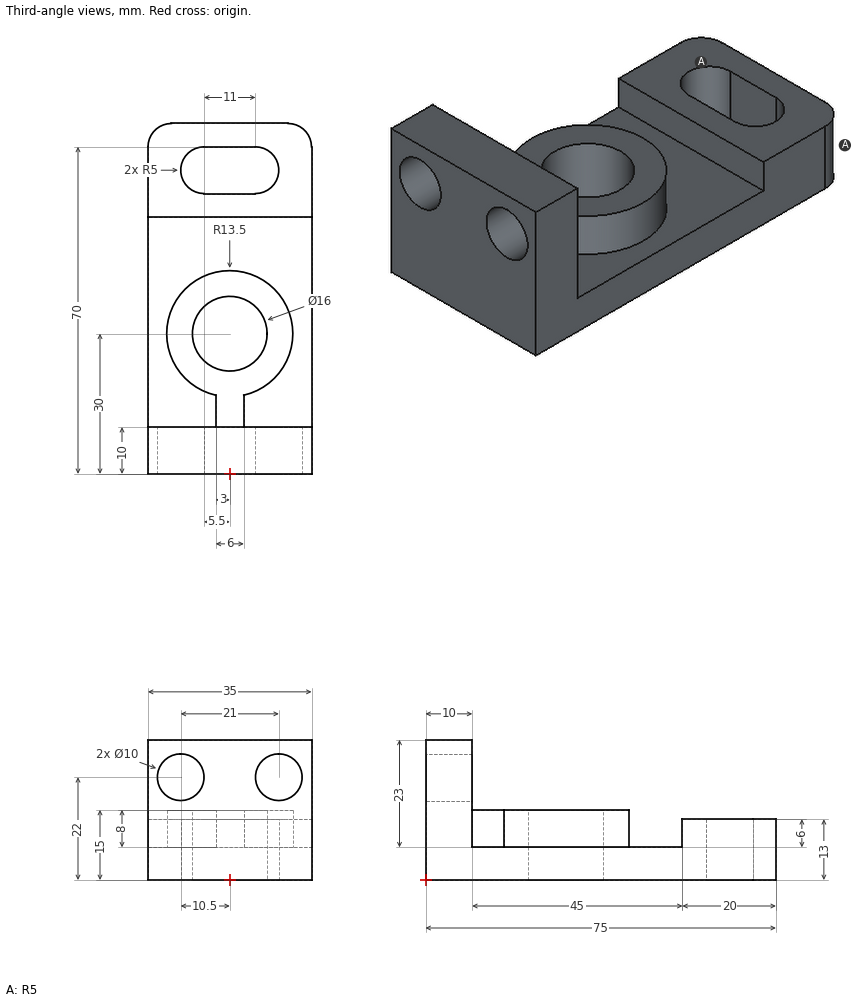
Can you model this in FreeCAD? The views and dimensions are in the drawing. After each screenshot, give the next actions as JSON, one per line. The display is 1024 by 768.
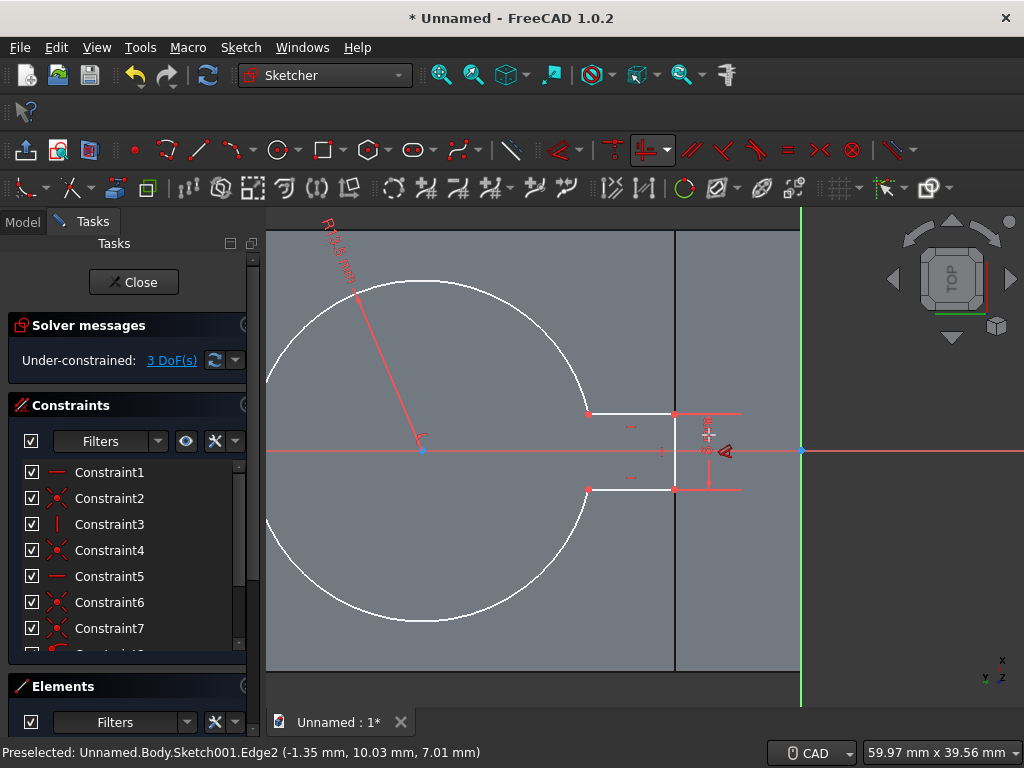
{"action": "left_click", "coordinate": [588, 490]}
{"action": "left_click", "coordinate": [835, 470]}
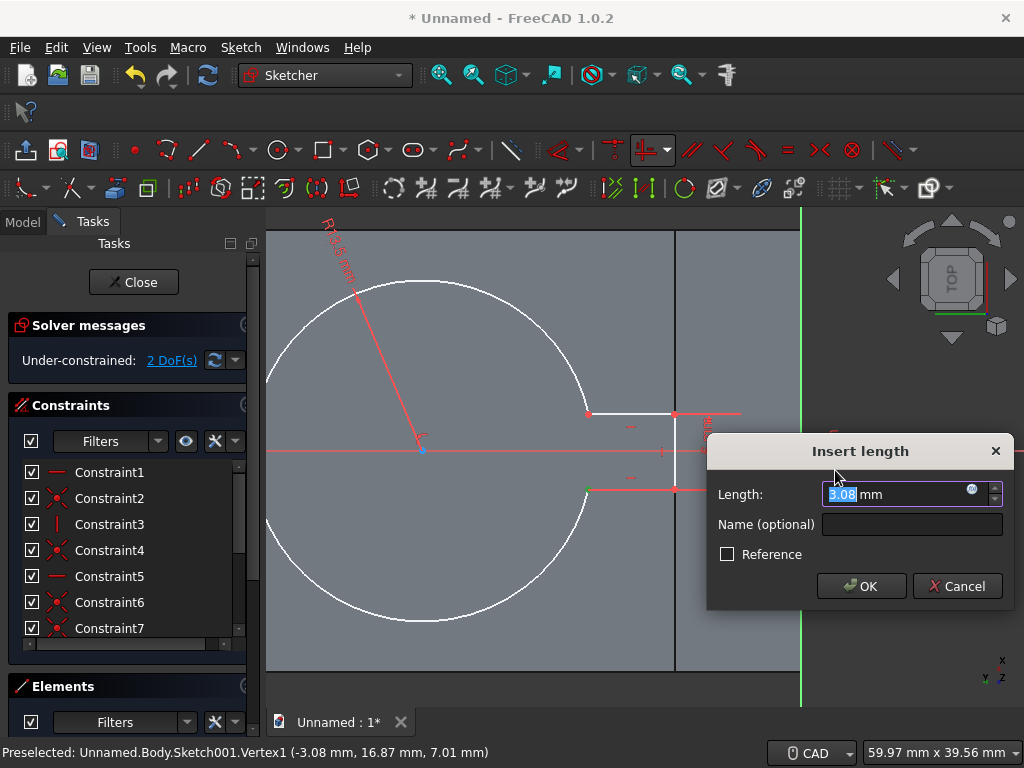
{"action": "type", "text": "3"}
{"action": "key", "text": "Return"}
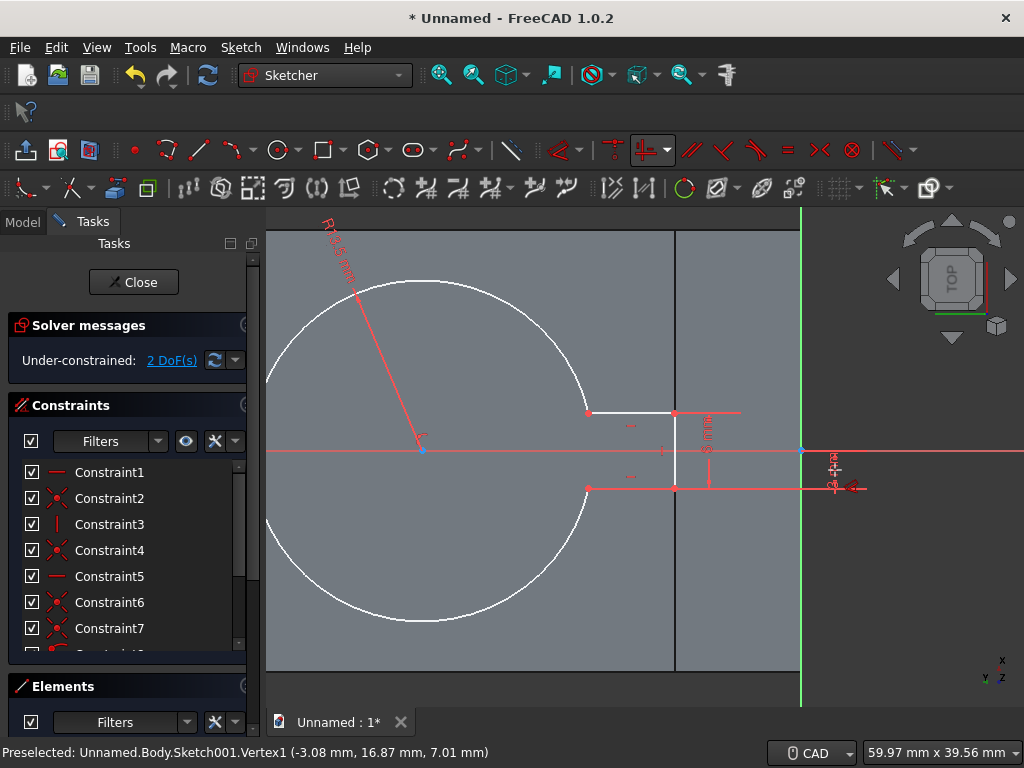
{"action": "left_click", "coordinate": [675, 489]}
{"action": "left_click", "coordinate": [738, 523]}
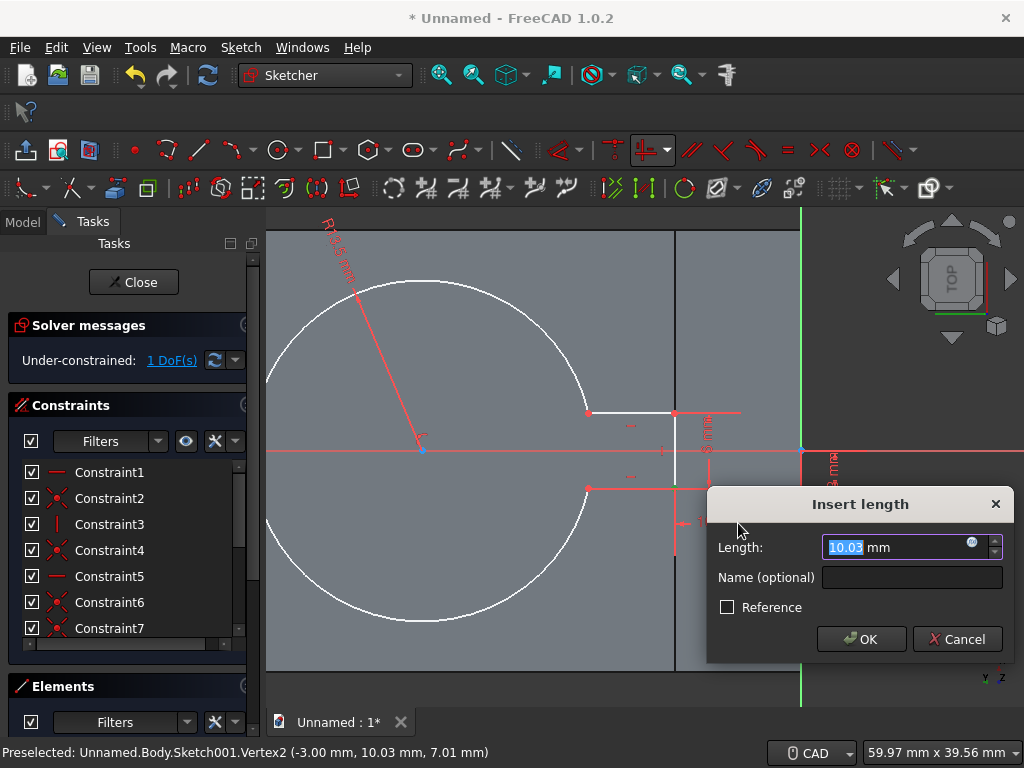
{"action": "type", "text": "10"}
{"action": "key", "text": "Return"}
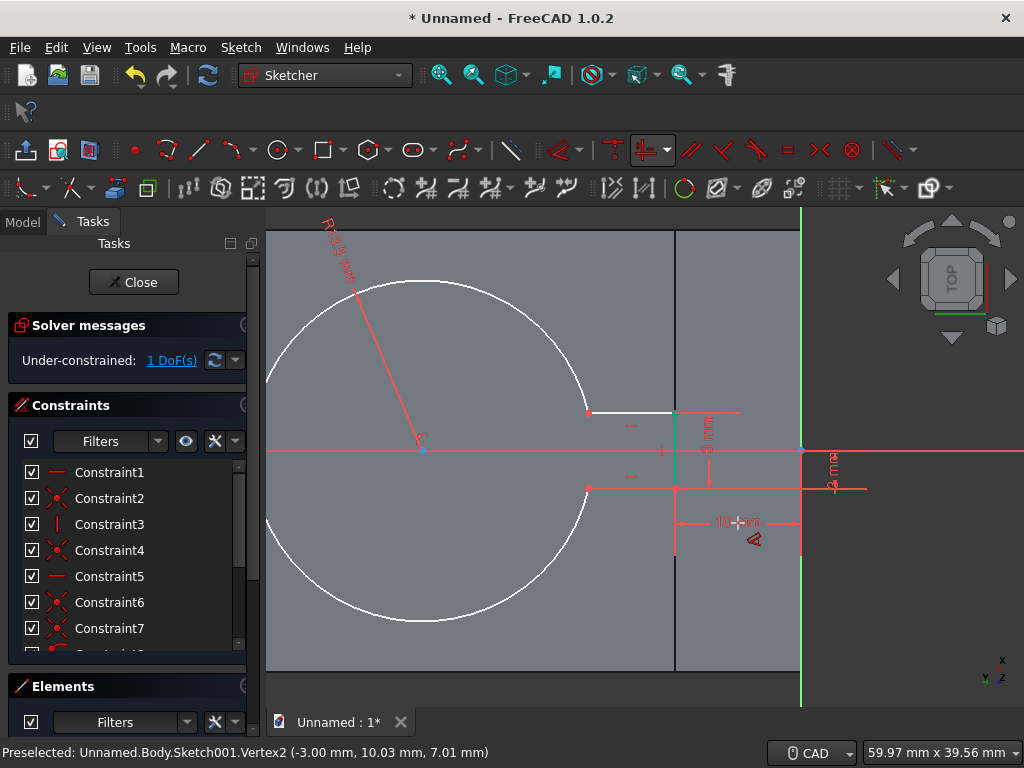
{"action": "left_click", "coordinate": [422, 451]}
{"action": "left_click", "coordinate": [525, 417]}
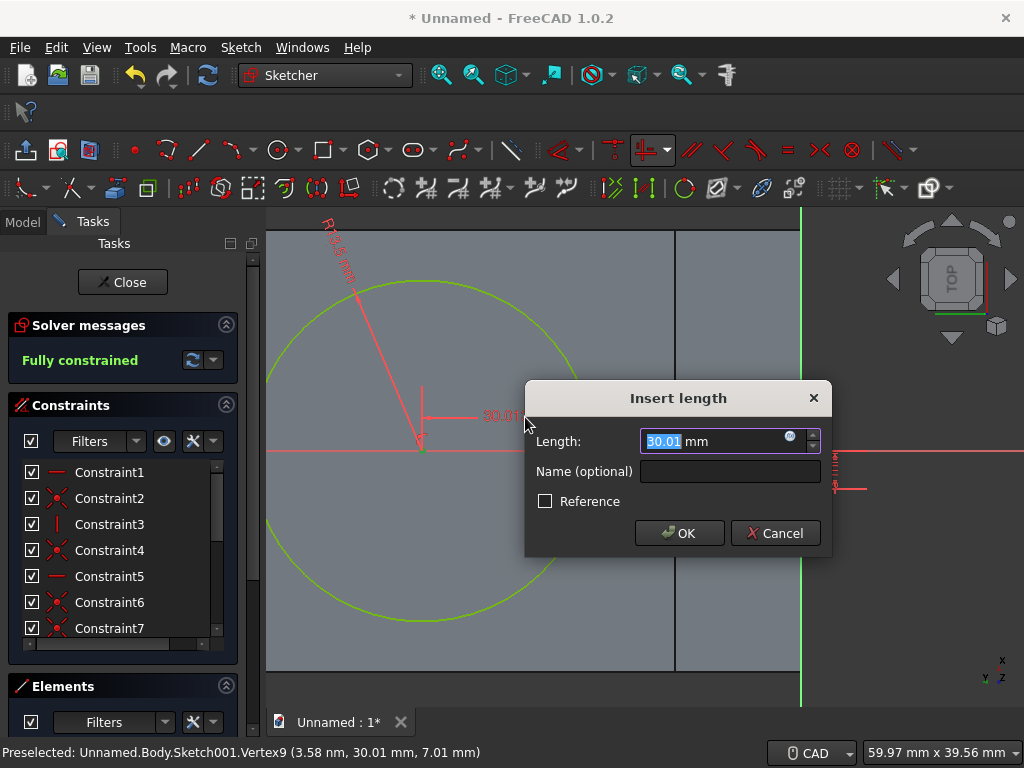
{"action": "type", "text": "30"}
{"action": "key", "text": "Return"}
{"action": "key", "text": "Escape"}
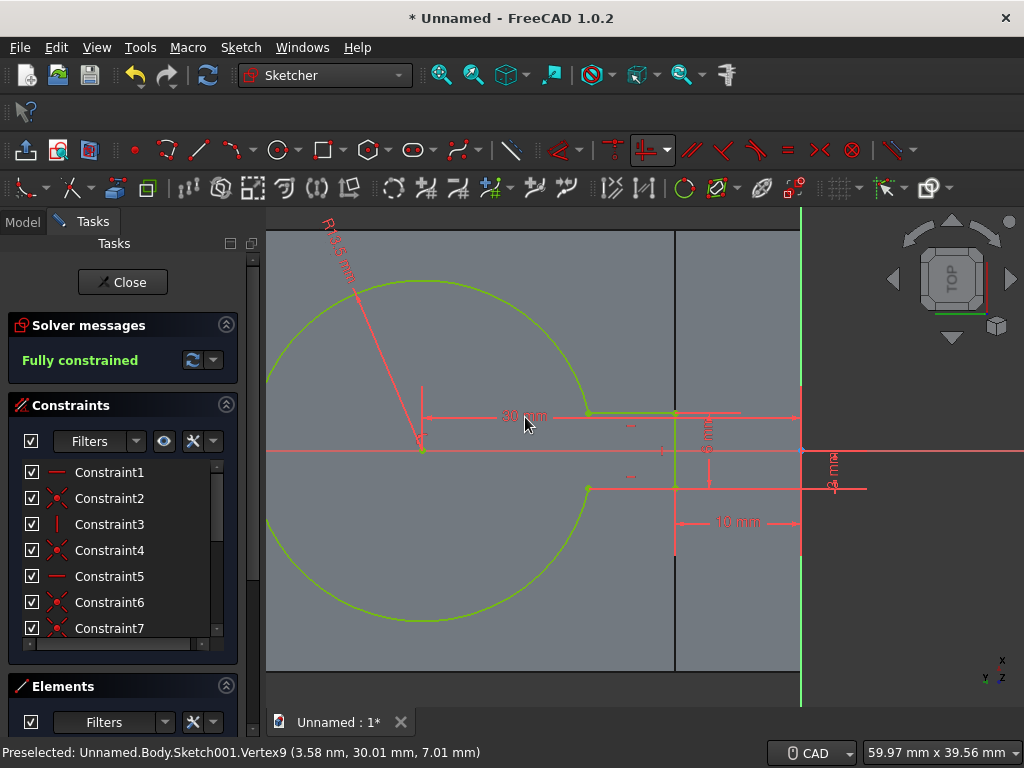
{"action": "left_click", "coordinate": [123, 282]}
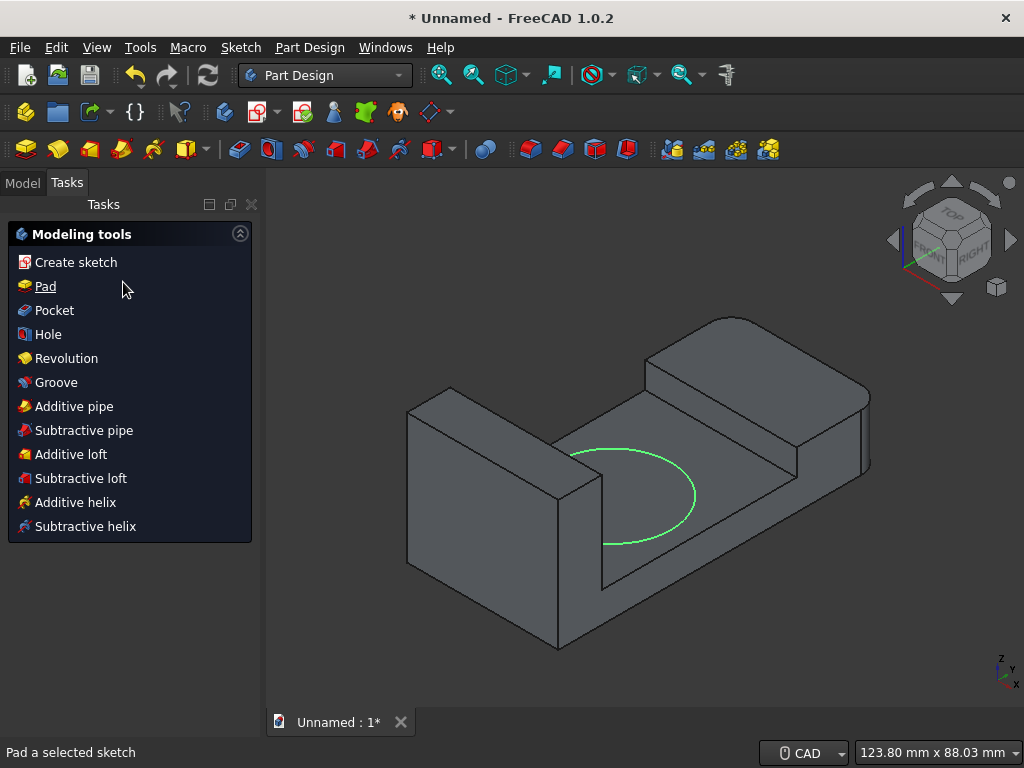
{"action": "left_click", "coordinate": [26, 150]}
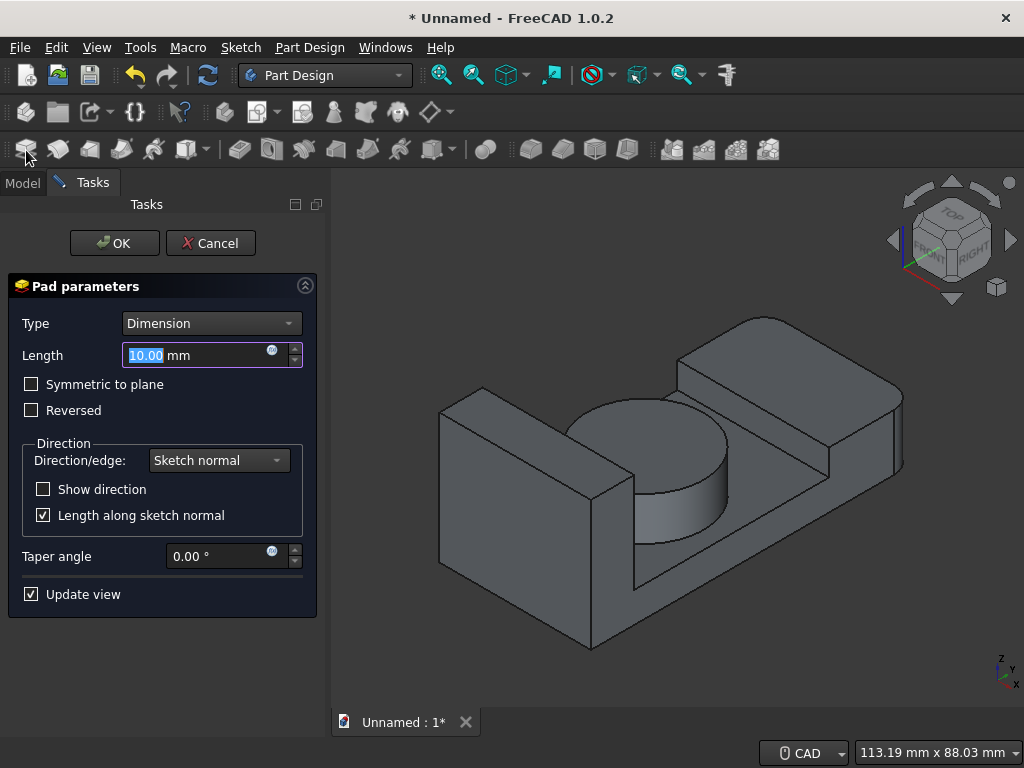
{"action": "type", "text": "8"}
{"action": "key", "text": "Tab"}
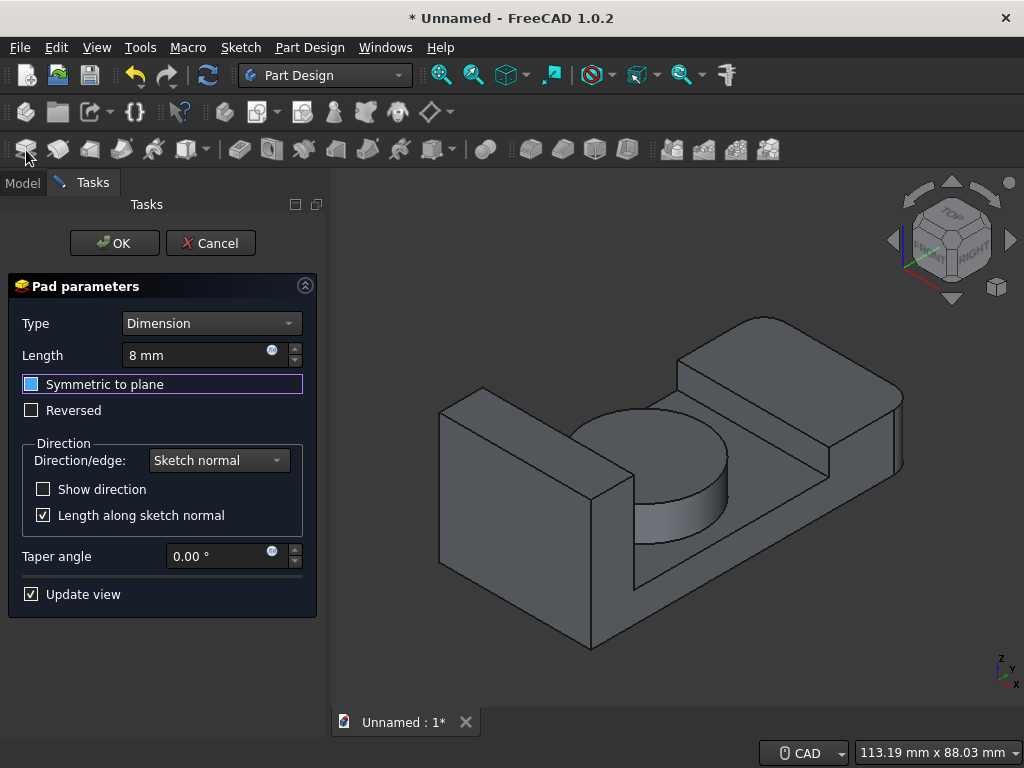
{"action": "left_click", "coordinate": [115, 243]}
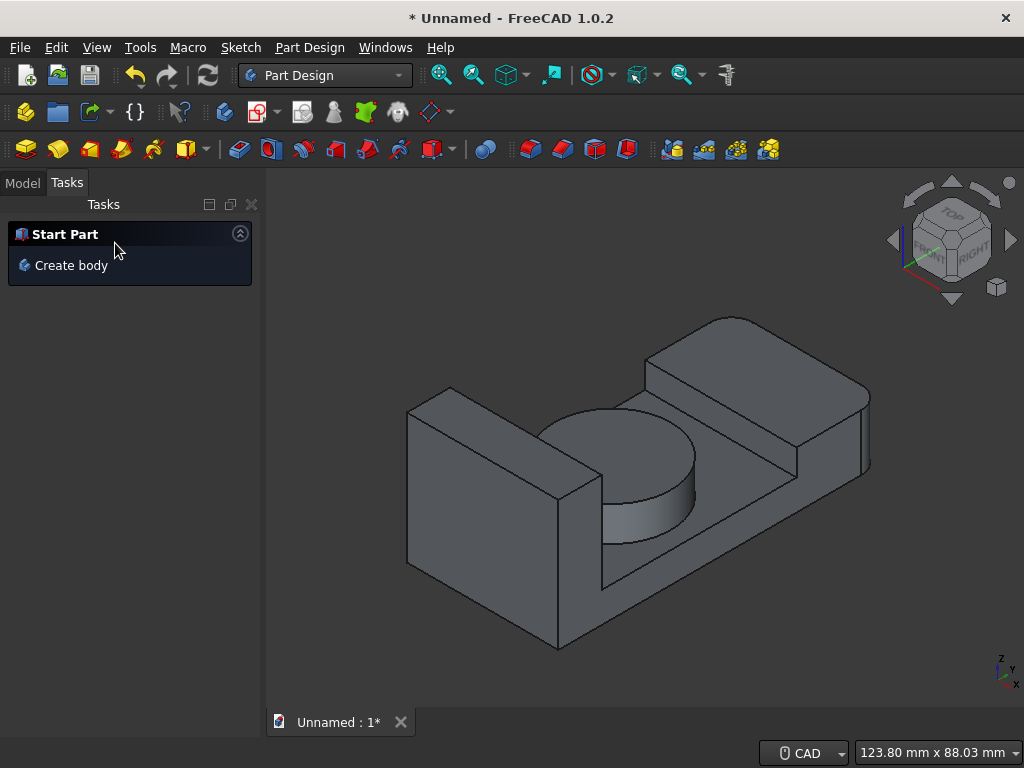
{"action": "left_click", "coordinate": [619, 451]}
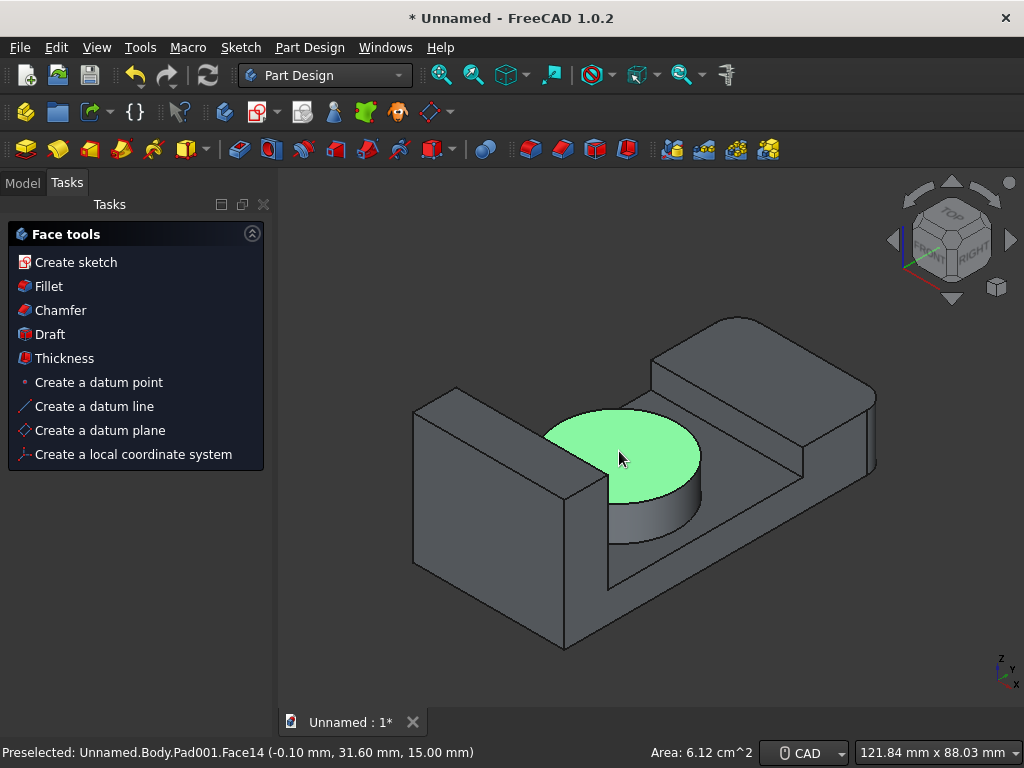
{"action": "left_click", "coordinate": [258, 112]}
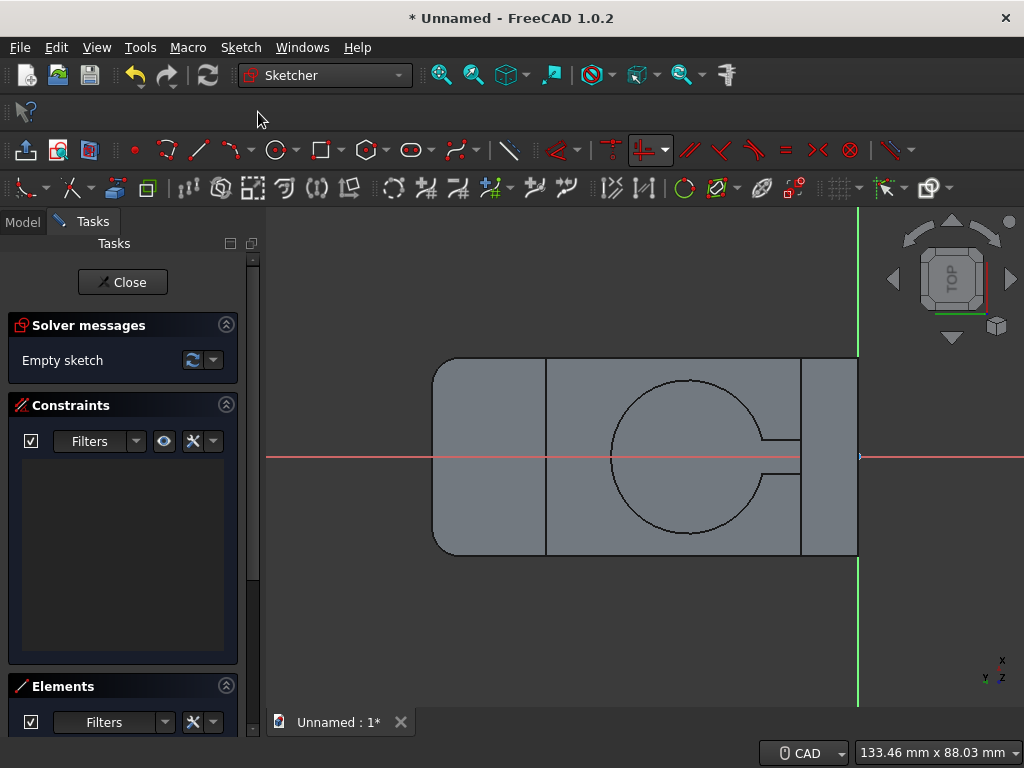
{"action": "key", "text": "q s"}